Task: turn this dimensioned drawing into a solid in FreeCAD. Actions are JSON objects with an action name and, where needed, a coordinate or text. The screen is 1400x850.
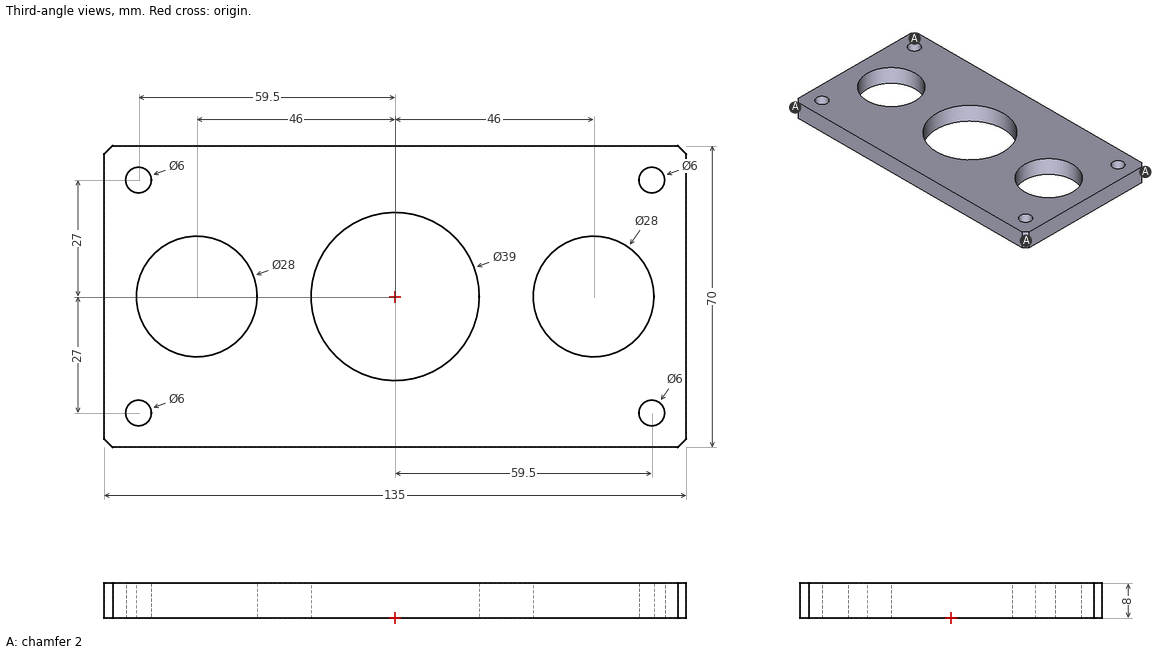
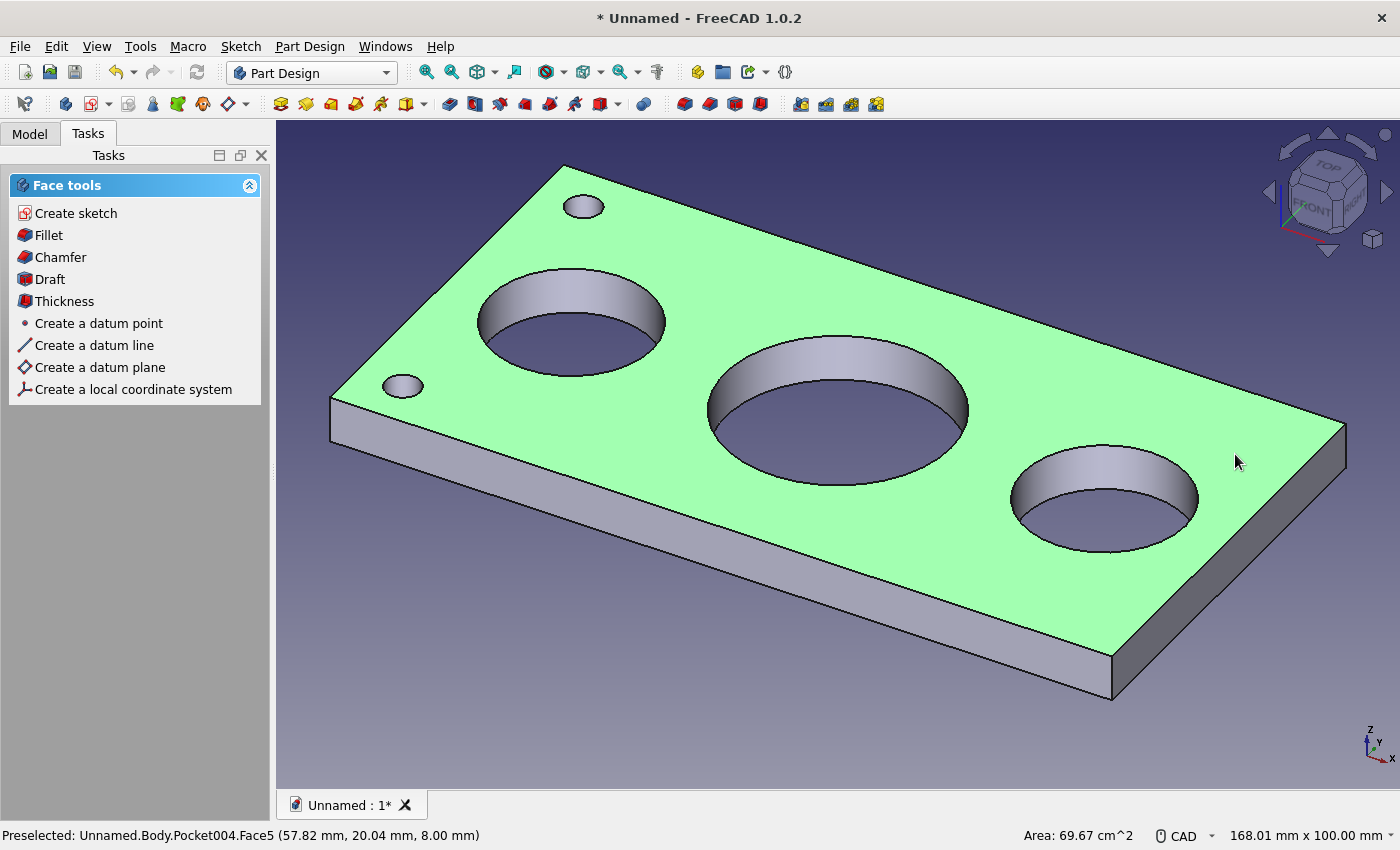
{"action": "left_click", "coordinate": [90, 104]}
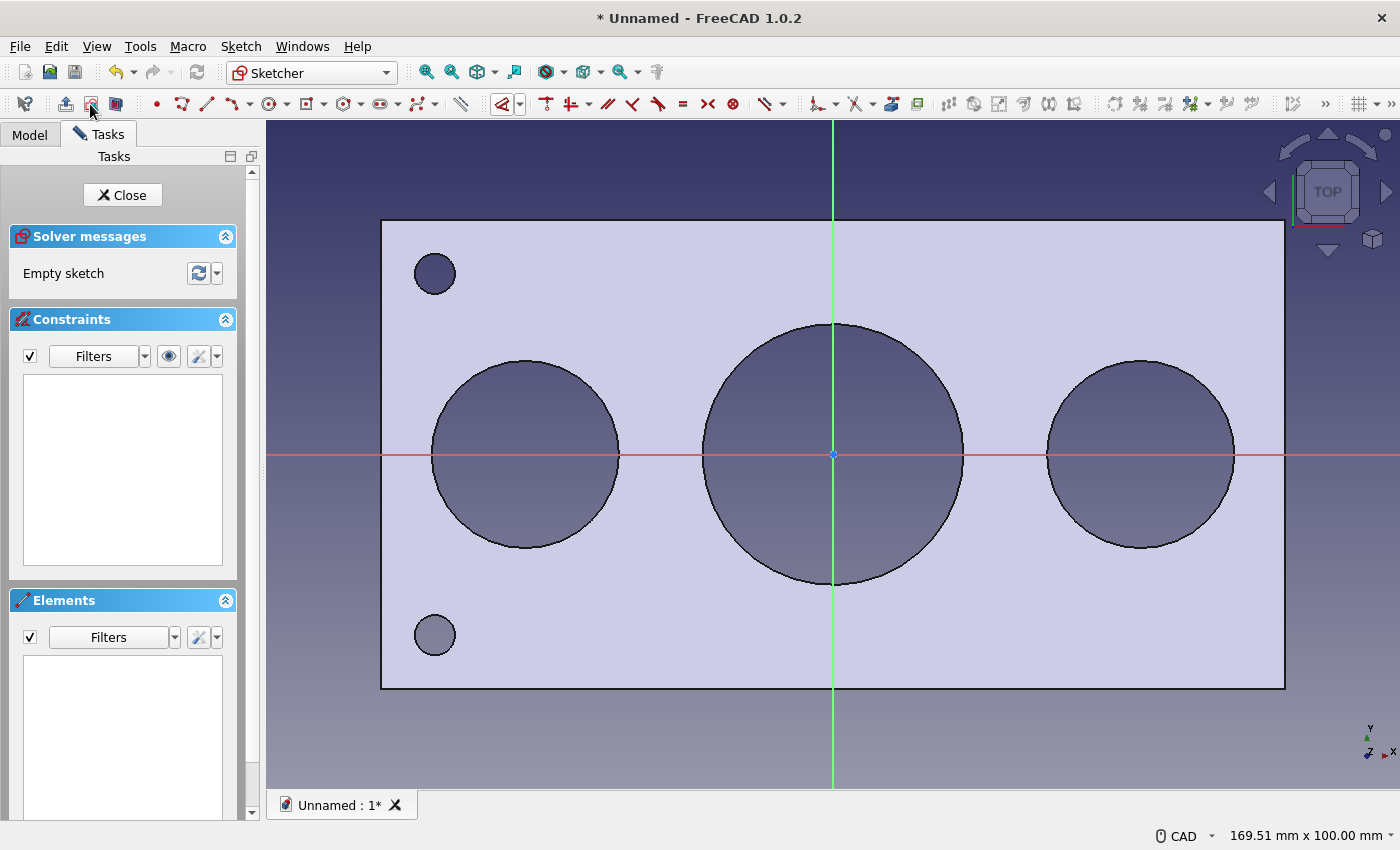
{"action": "scroll", "coordinate": [764, 454], "scroll_direction": "down", "scroll_amount": 5}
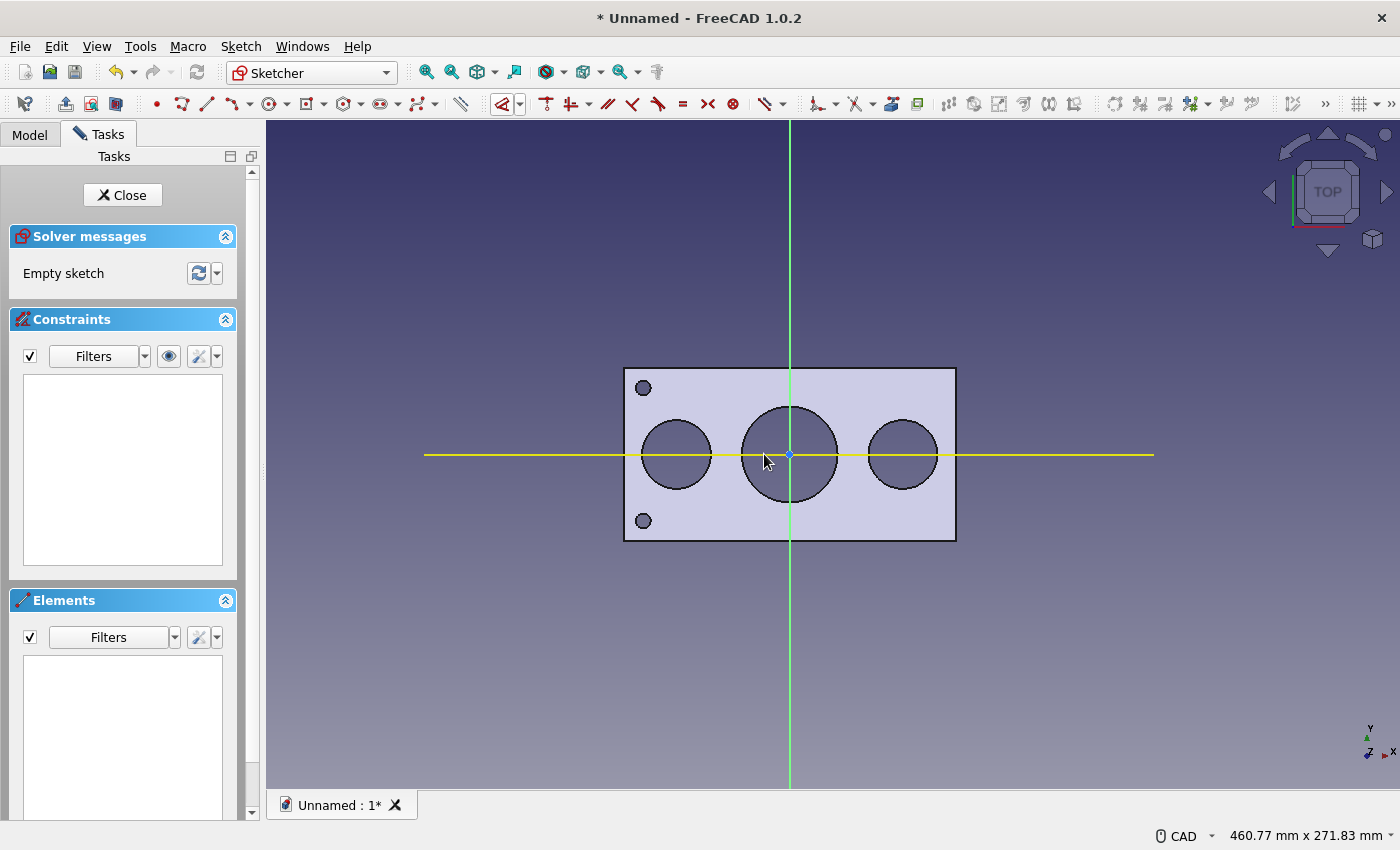
{"action": "scroll", "coordinate": [945, 524], "scroll_direction": "up", "scroll_amount": 15}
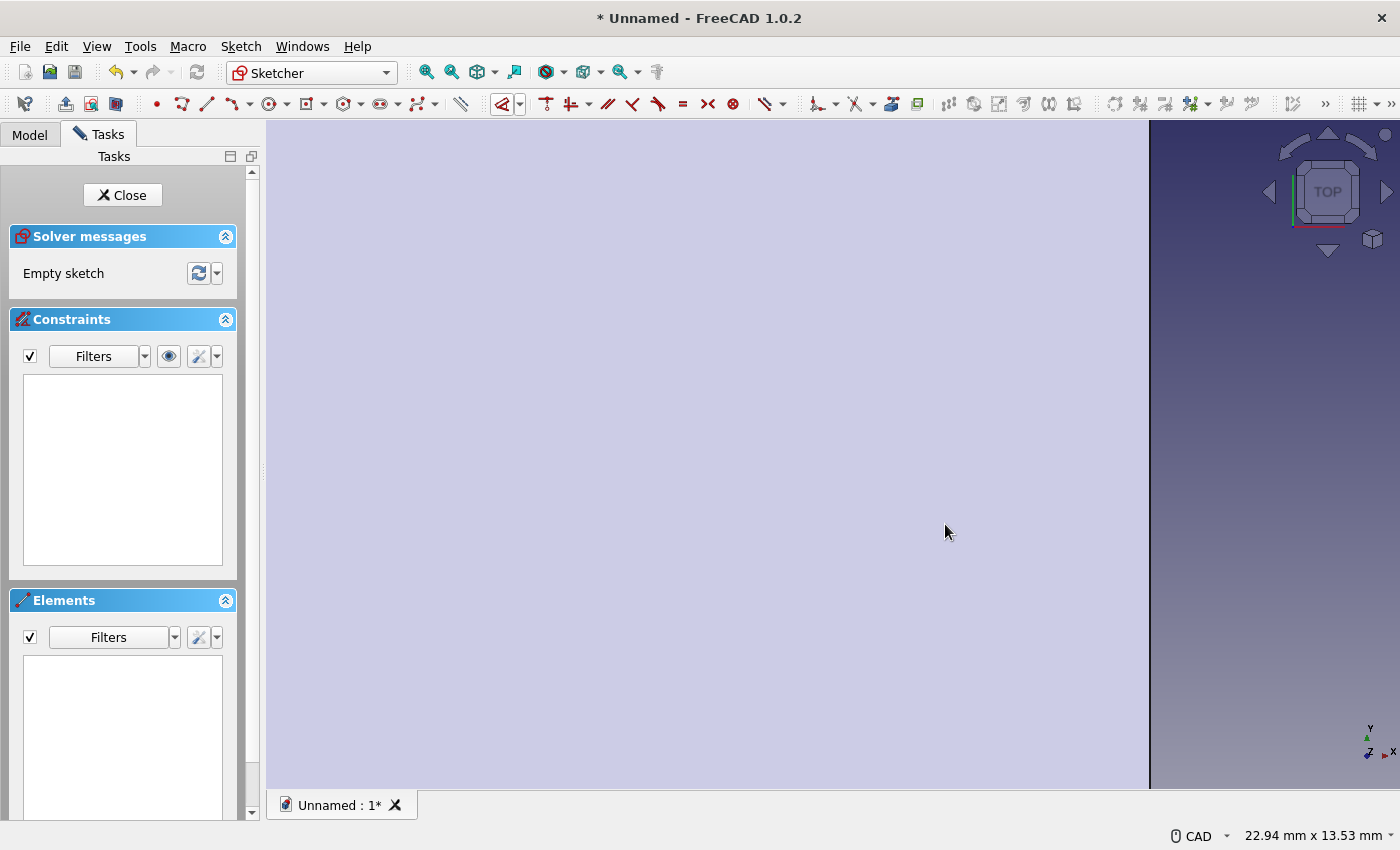
{"action": "scroll", "coordinate": [735, 444], "scroll_direction": "up", "scroll_amount": 2}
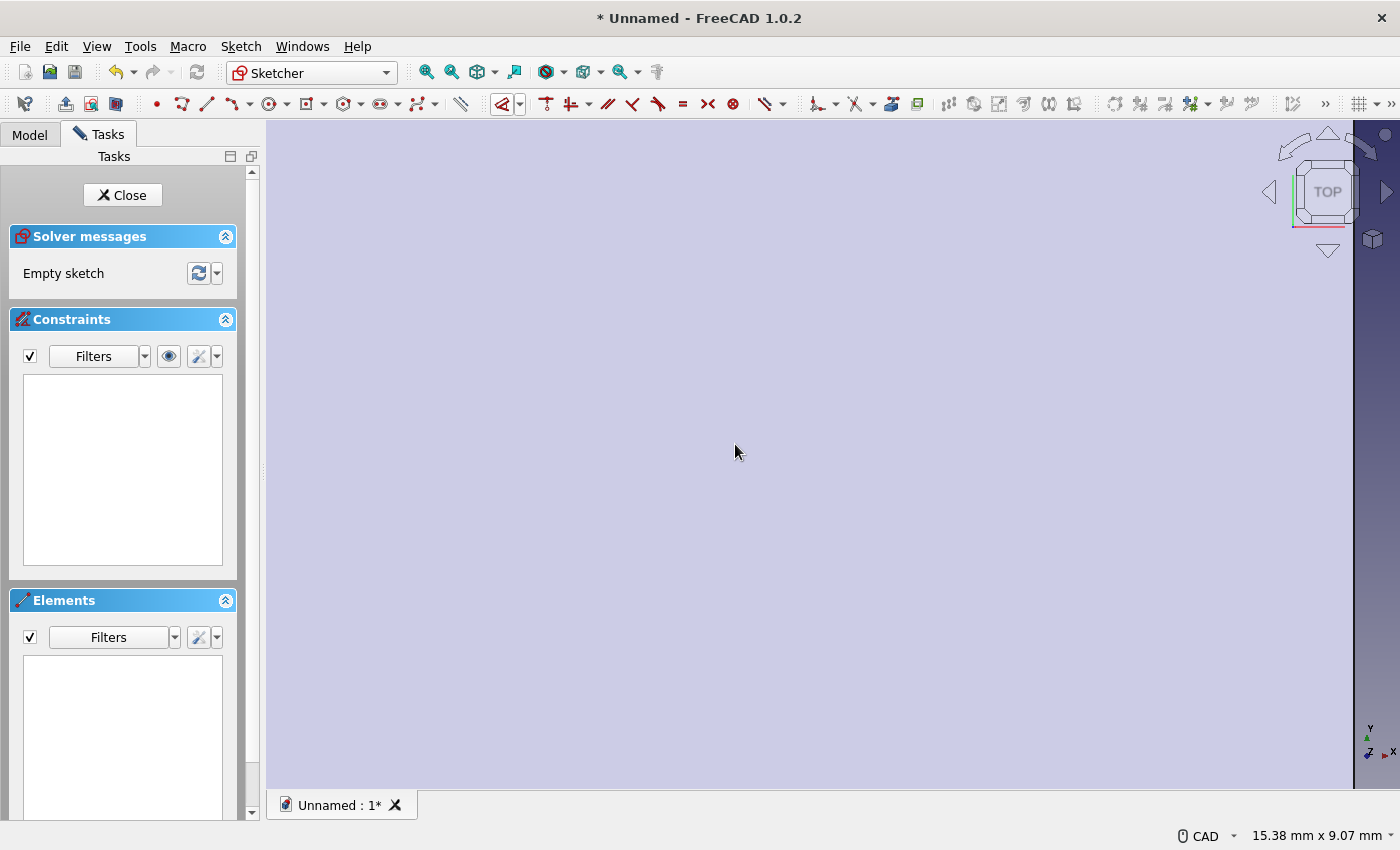
{"action": "key", "text": "g c"}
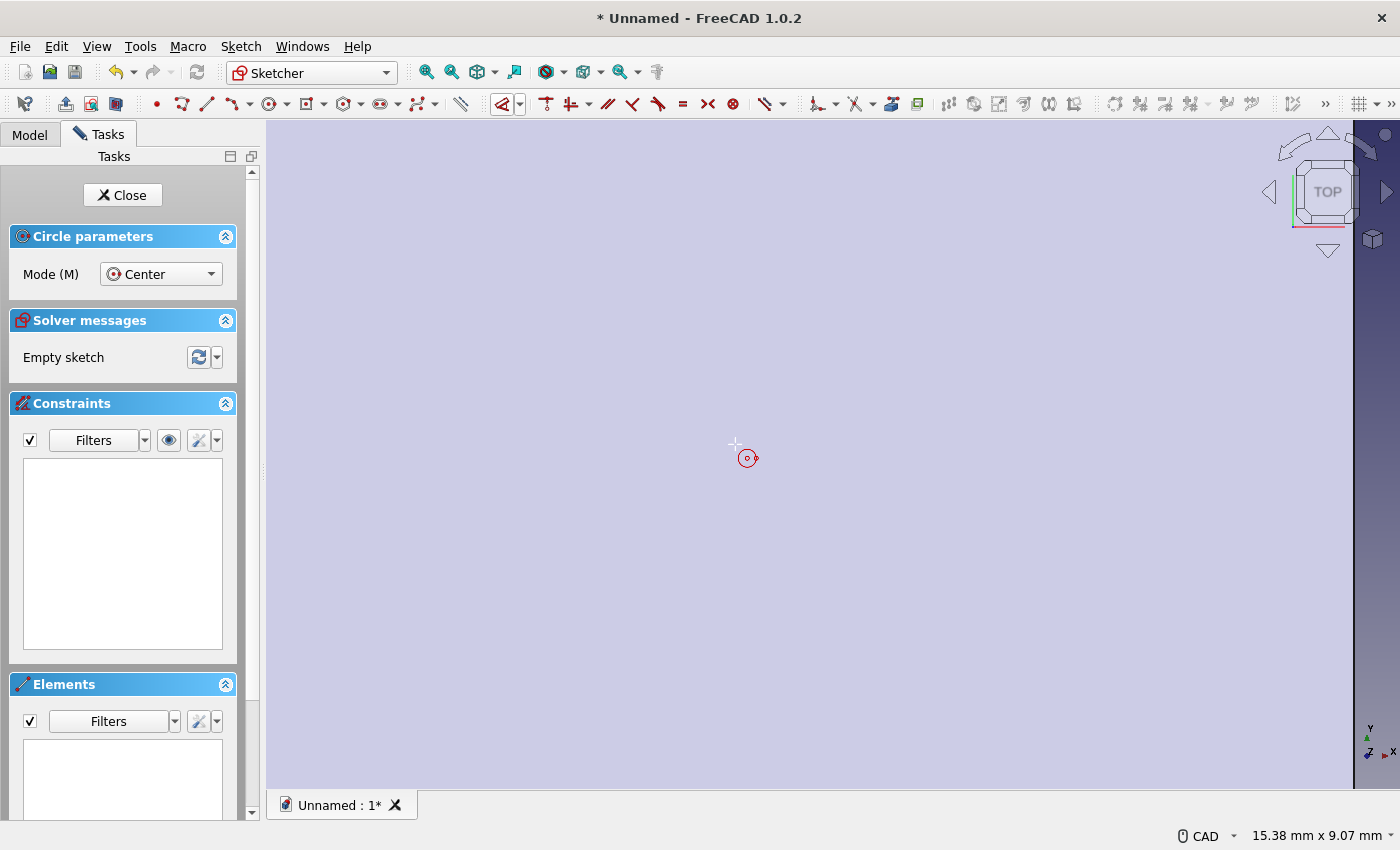
{"action": "left_click", "coordinate": [764, 454]}
{"action": "left_click", "coordinate": [921, 298]}
{"action": "key", "text": "Escape"}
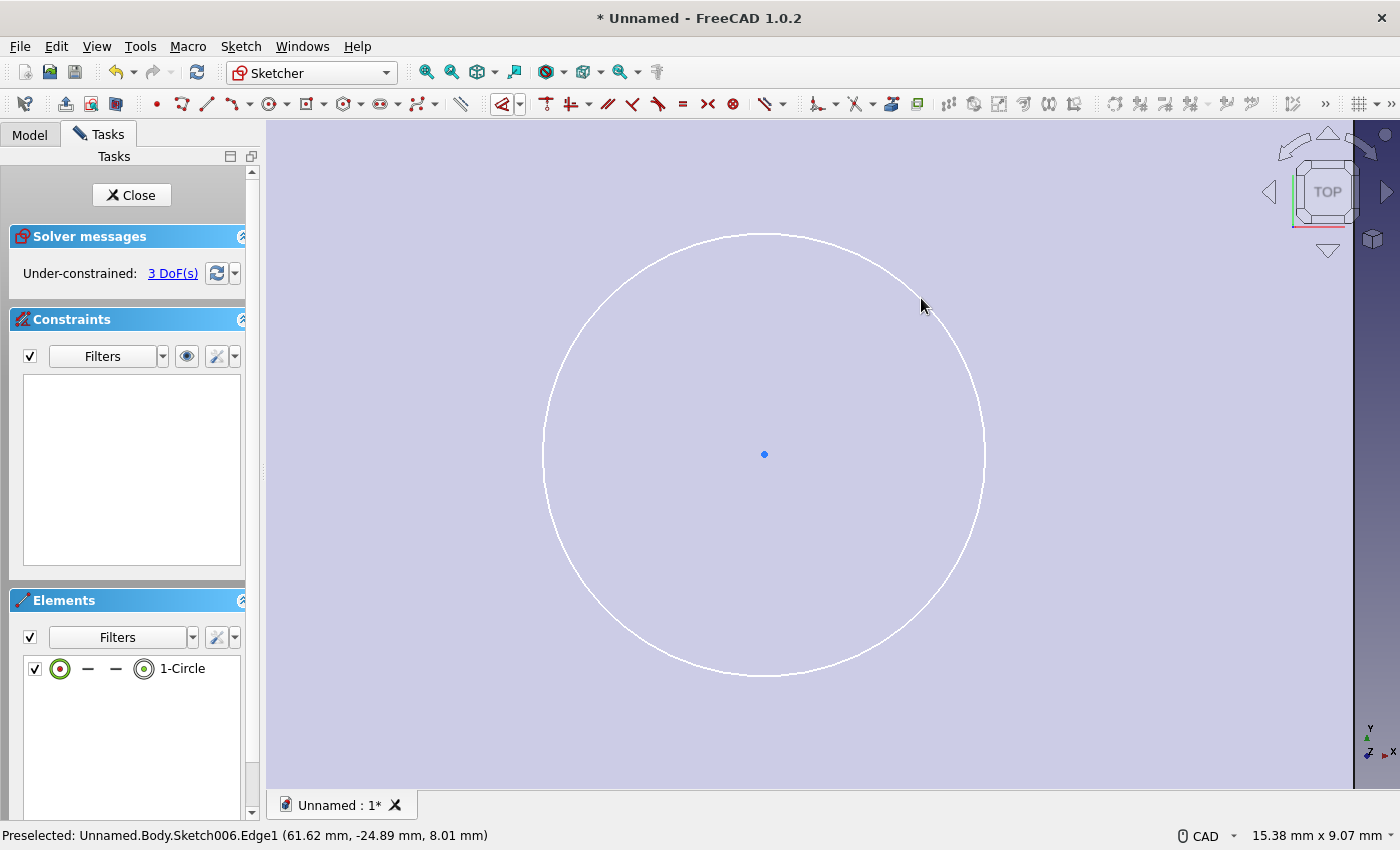
{"action": "left_click", "coordinate": [920, 298]}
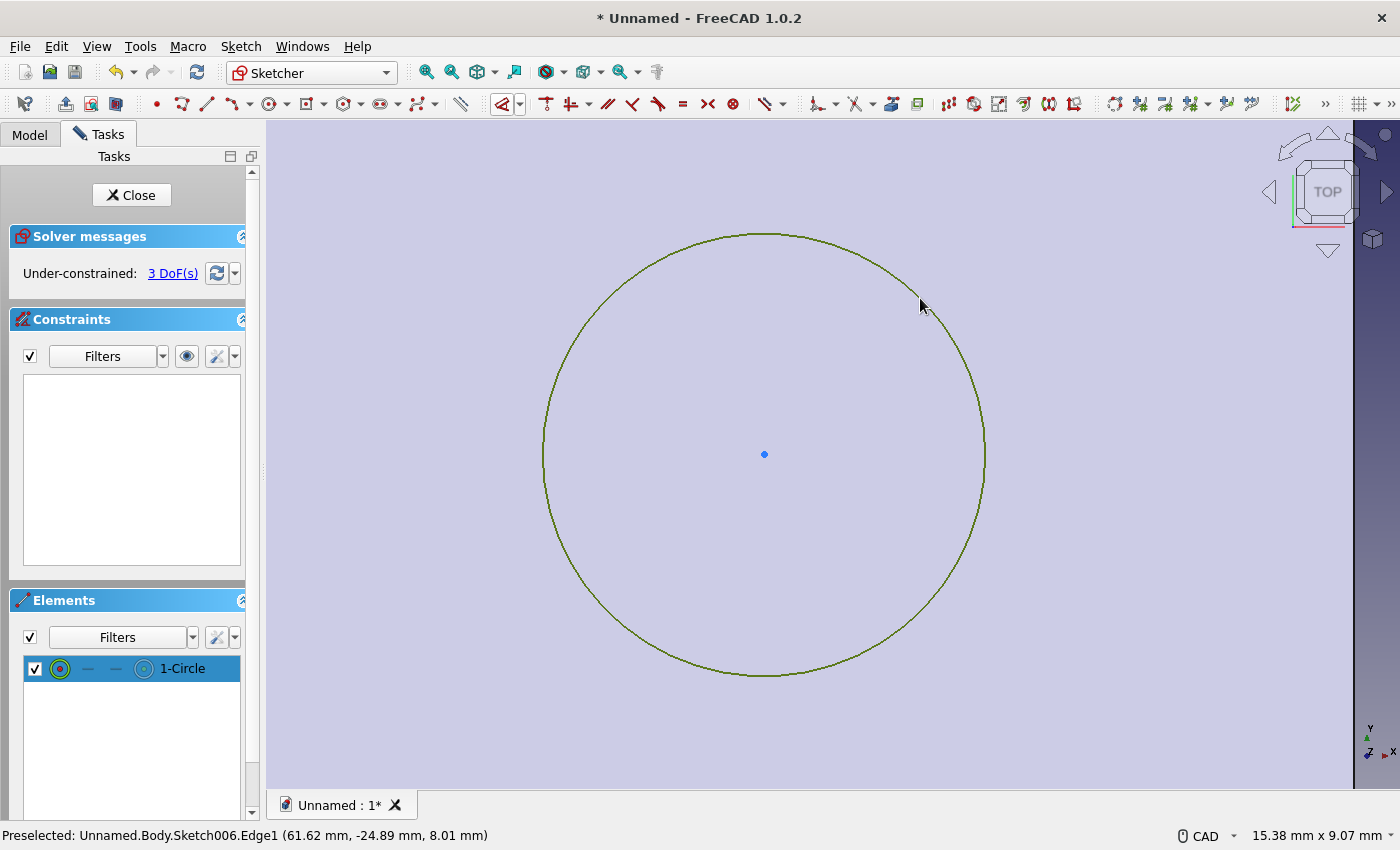
{"action": "left_click", "coordinate": [520, 104]}